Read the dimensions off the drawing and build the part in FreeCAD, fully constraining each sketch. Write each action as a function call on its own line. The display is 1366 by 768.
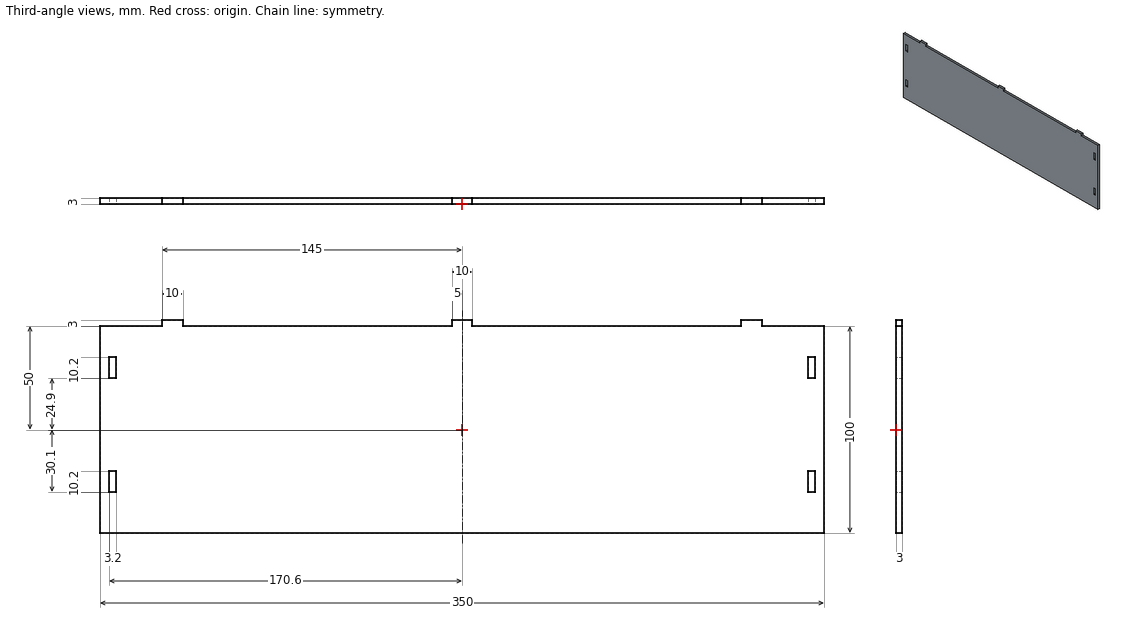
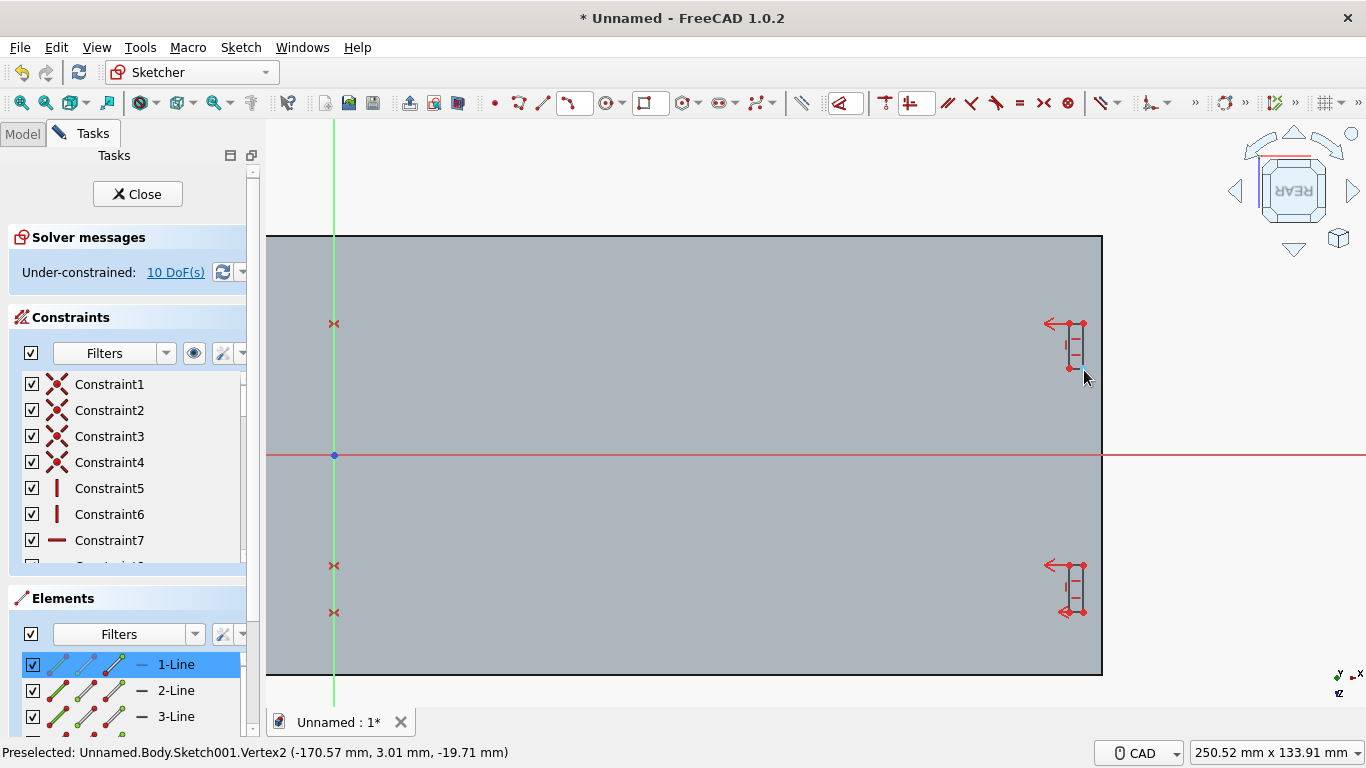
click(1083, 369)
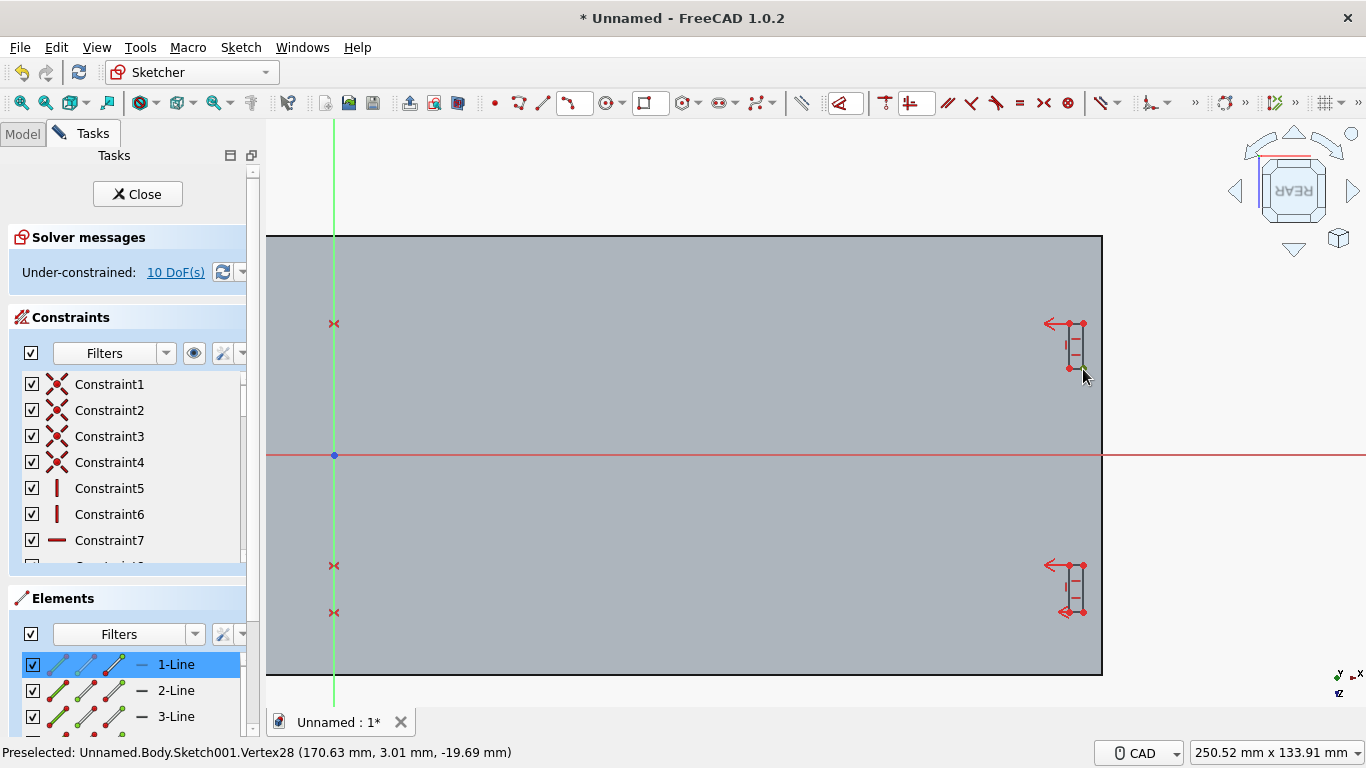
click(334, 641)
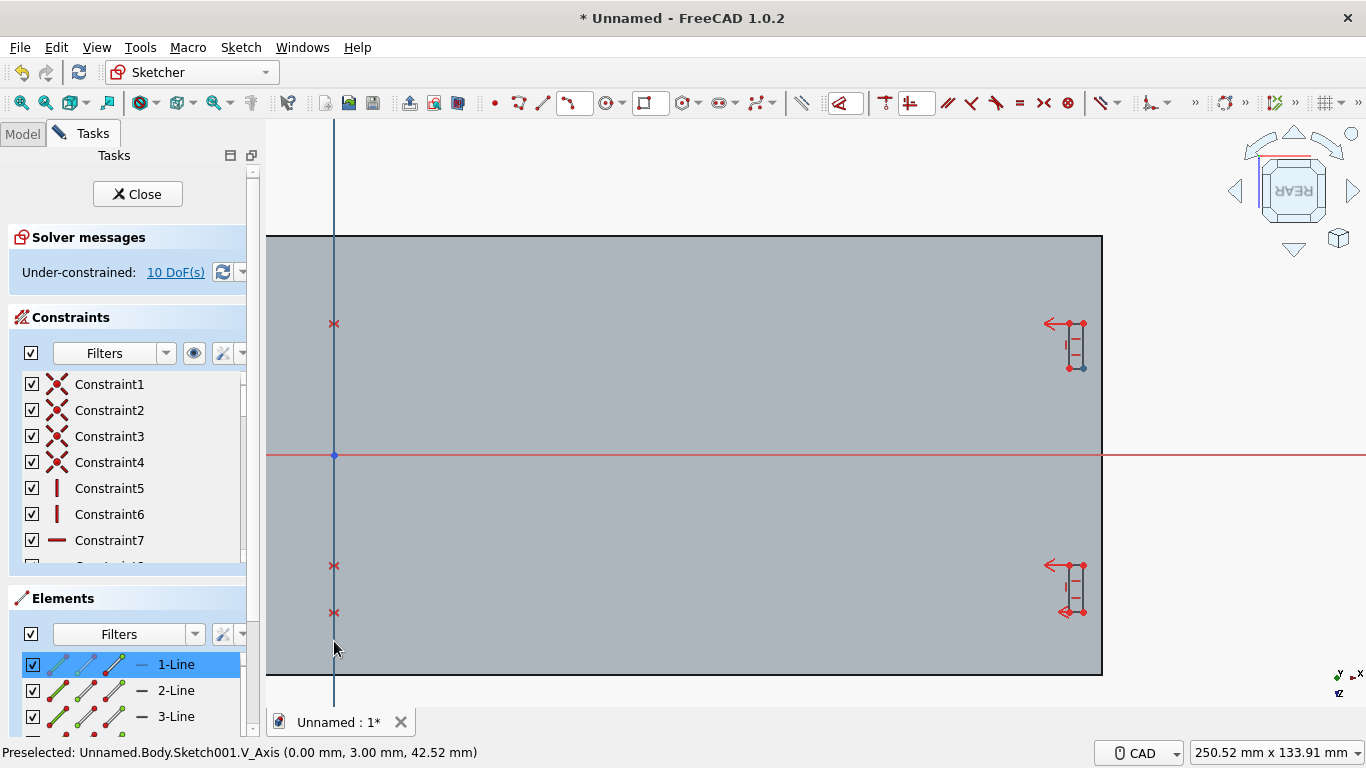
click(1044, 104)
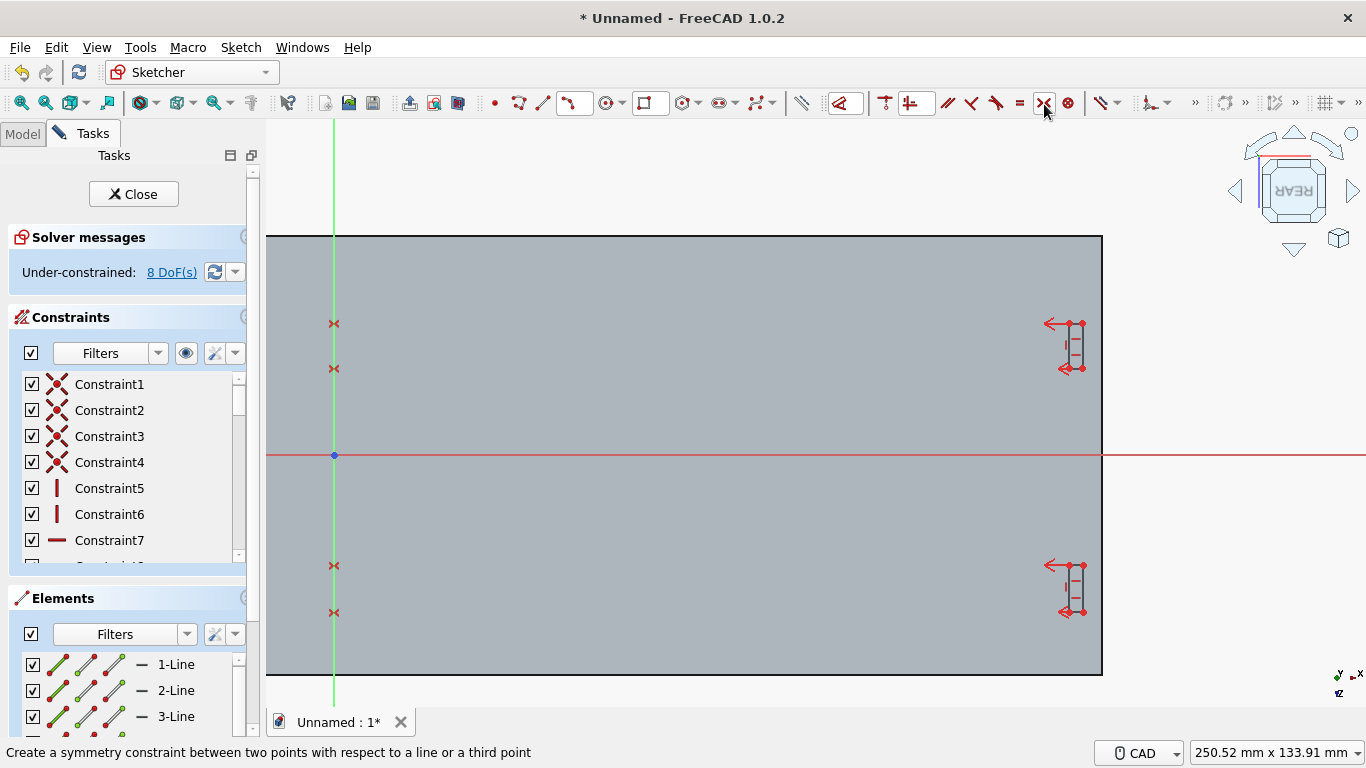
key(d)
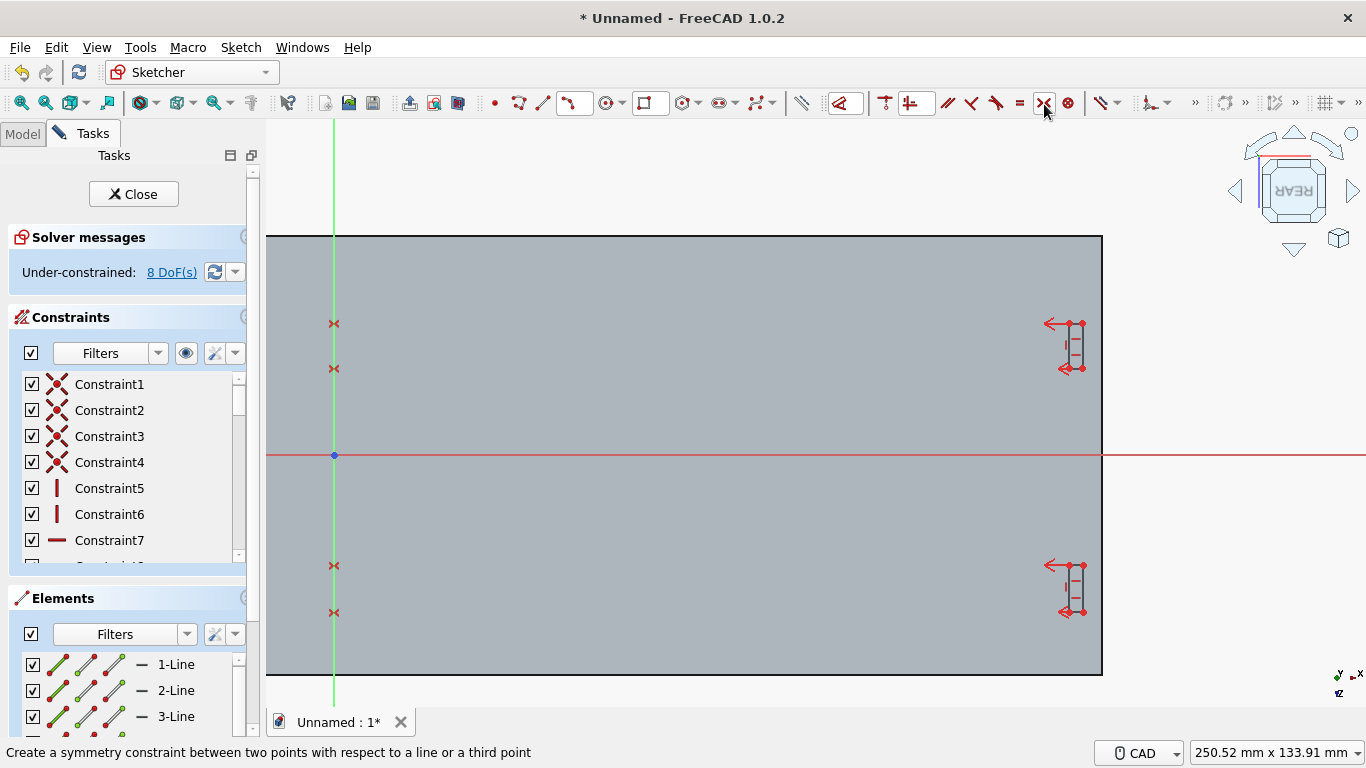
scroll(1085, 370, down, 4)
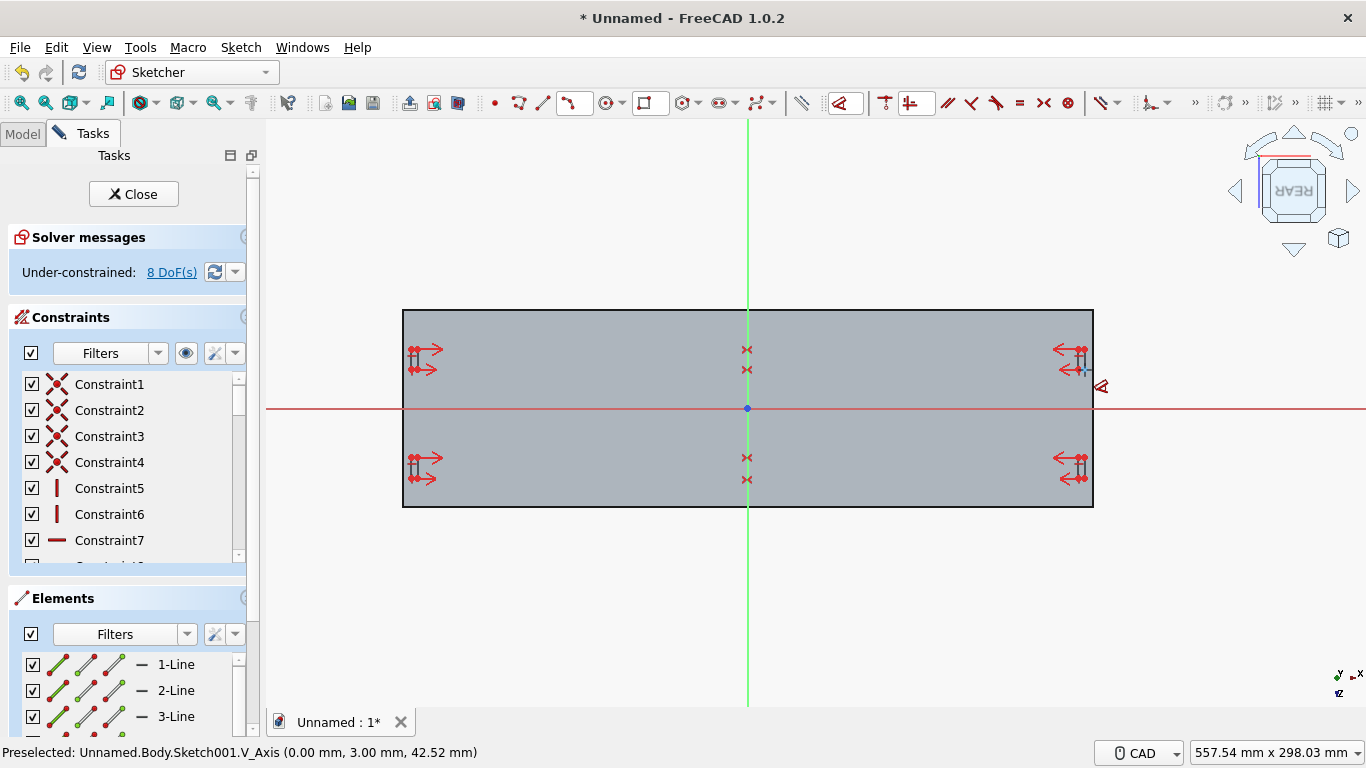
scroll(415, 370, up, 10)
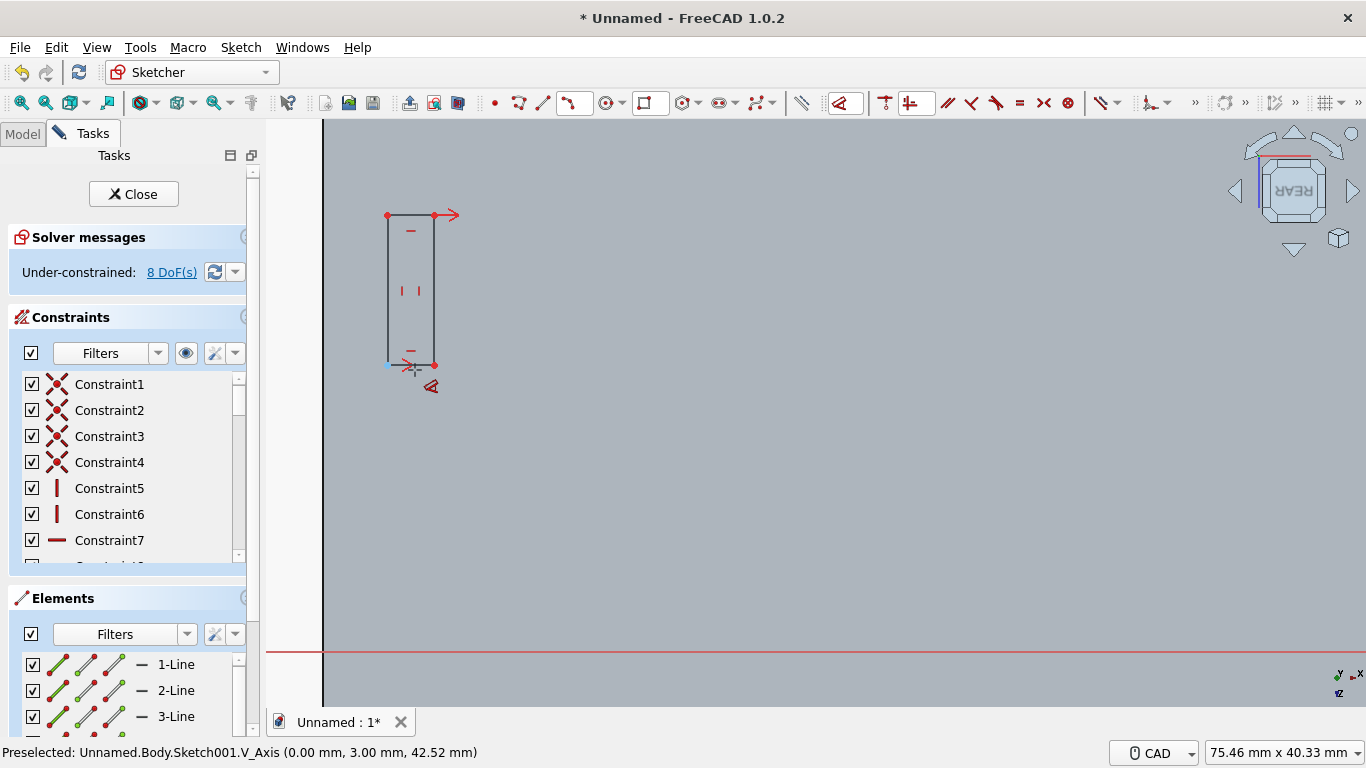
click(411, 365)
click(411, 331)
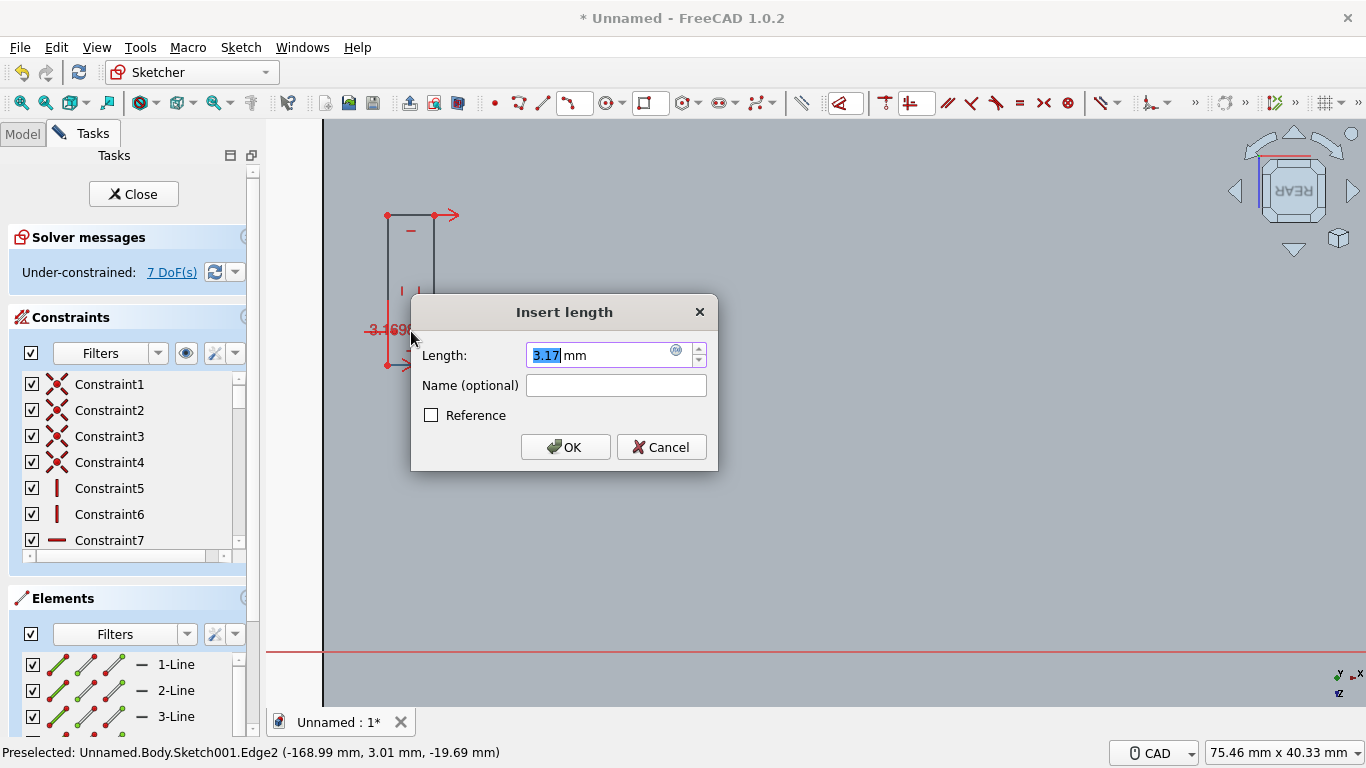
text(3.2)
key(Return)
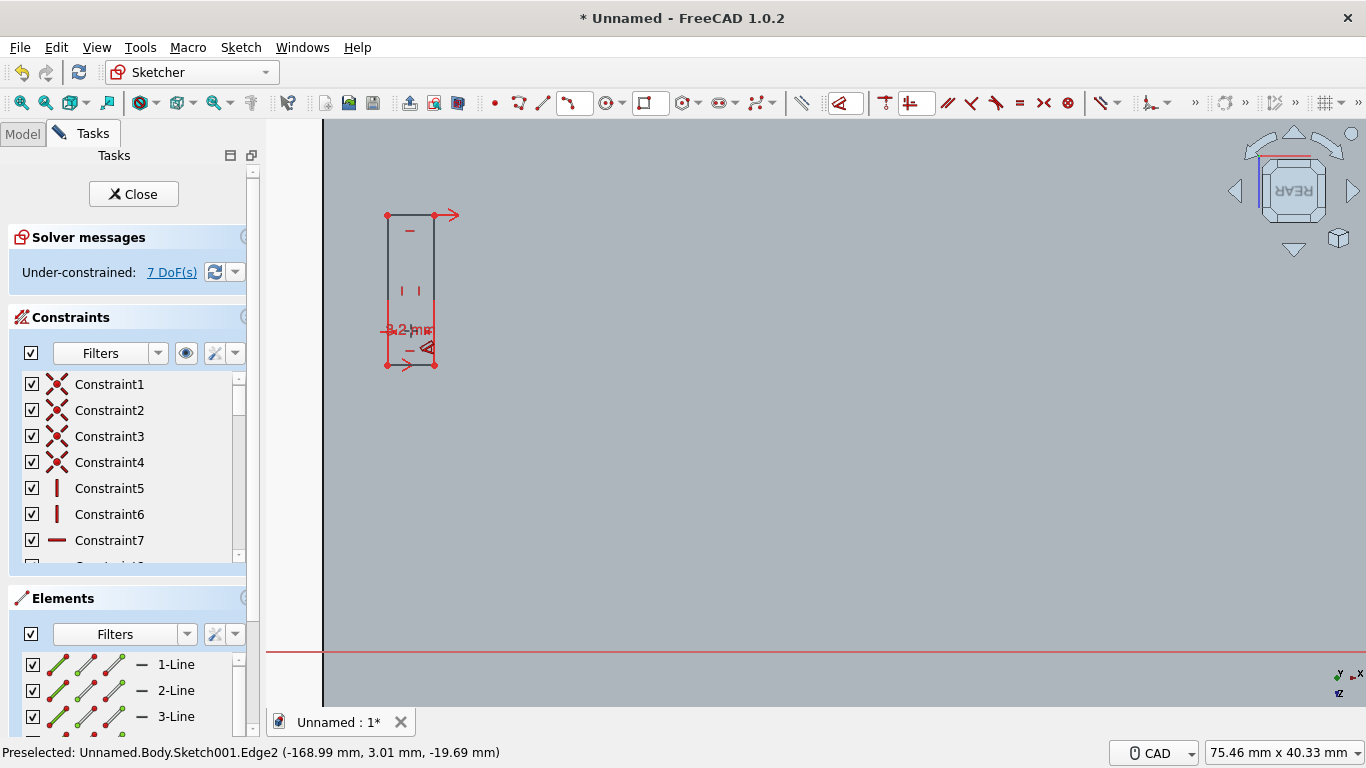
scroll(415, 370, down, 10)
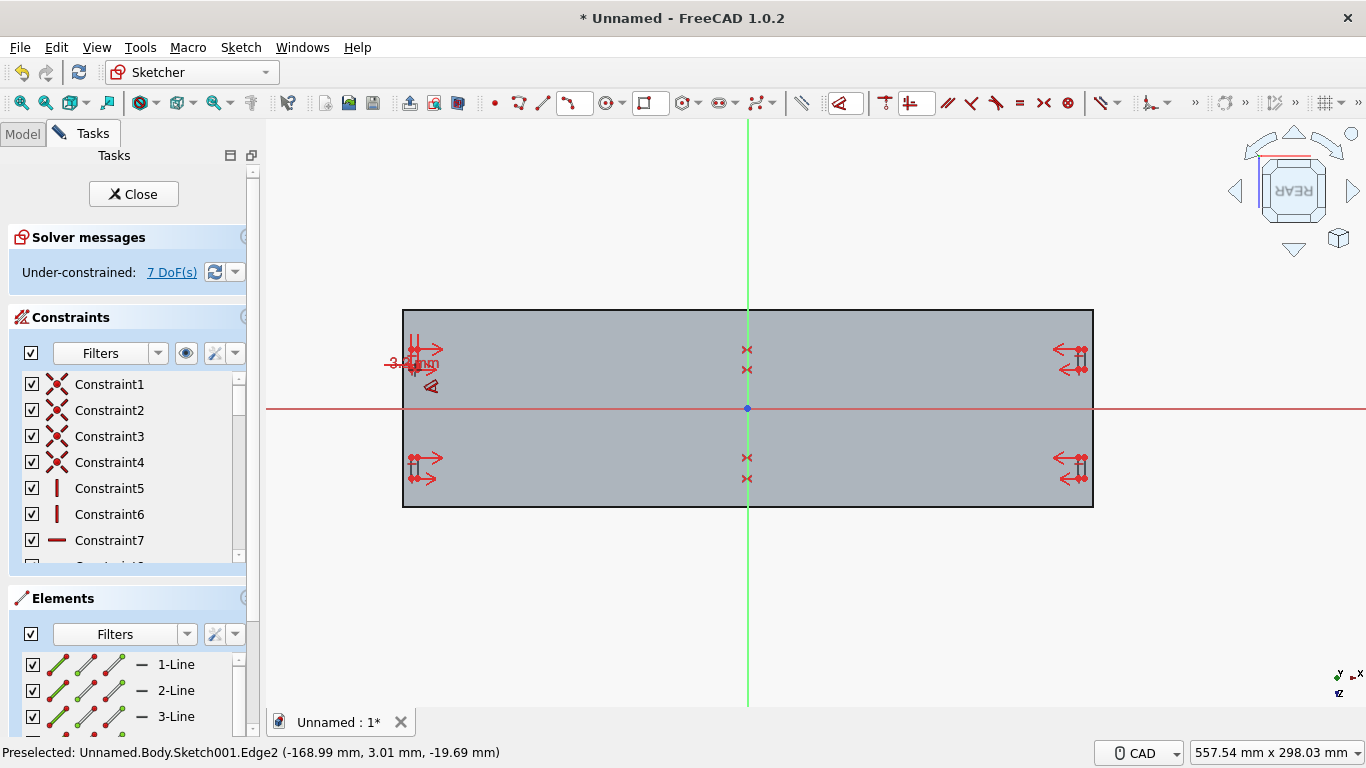
scroll(413, 479, up, 11)